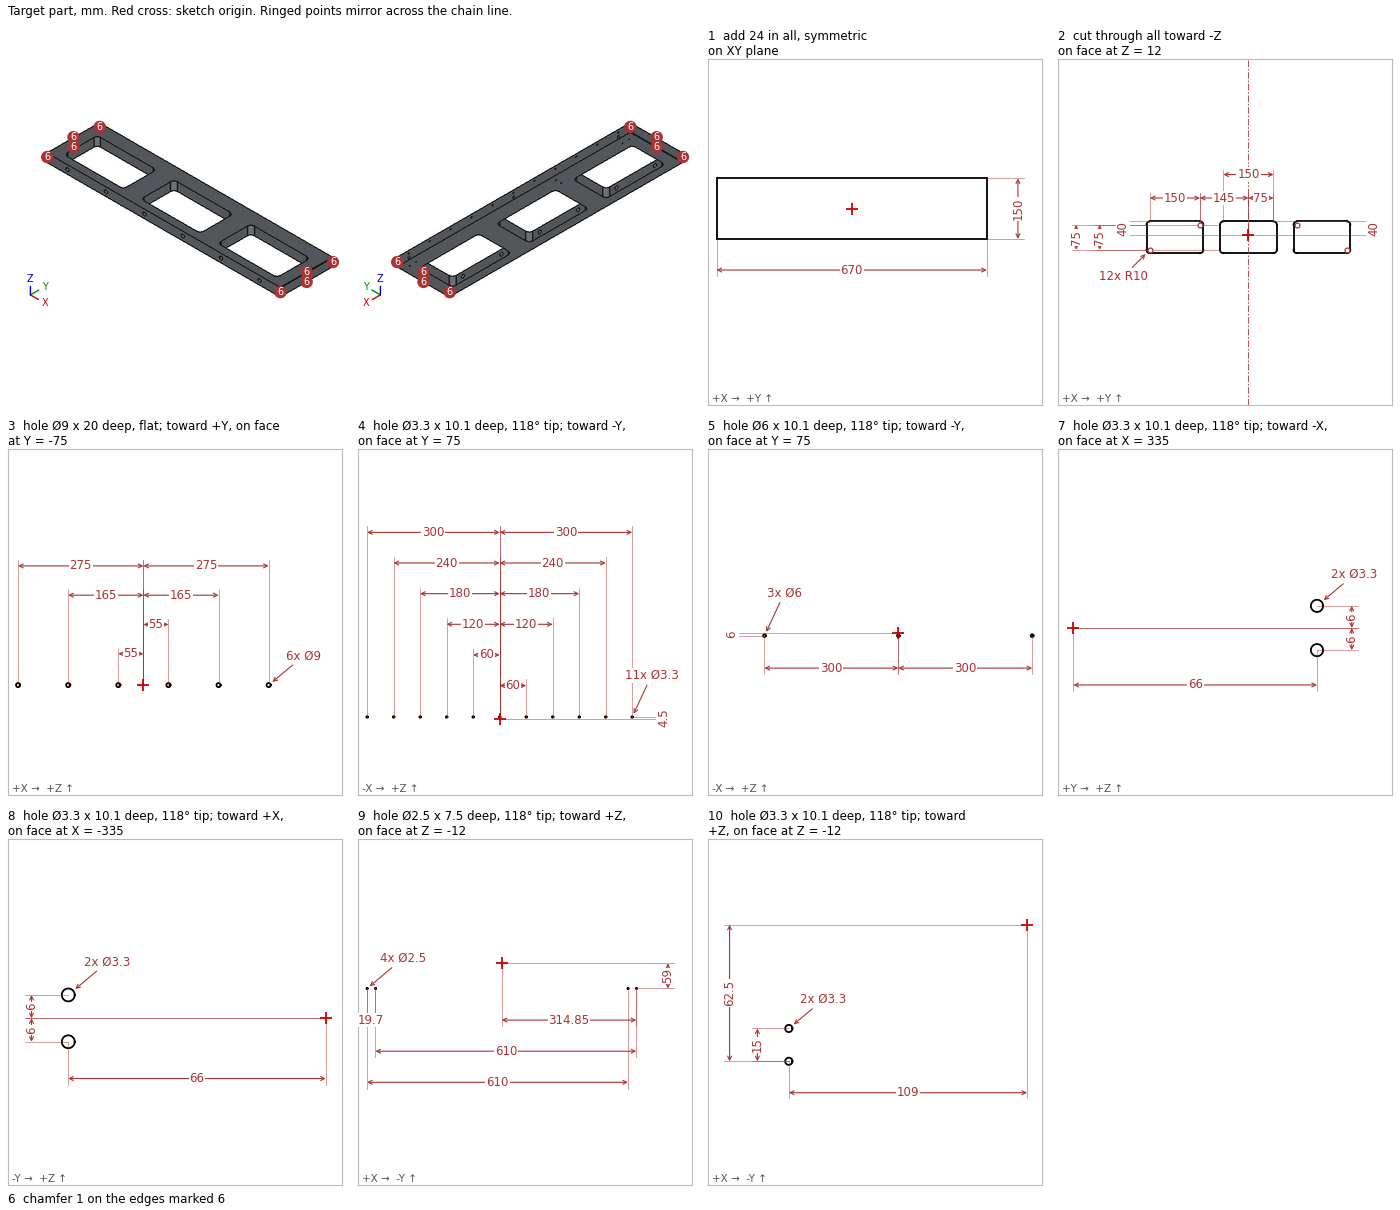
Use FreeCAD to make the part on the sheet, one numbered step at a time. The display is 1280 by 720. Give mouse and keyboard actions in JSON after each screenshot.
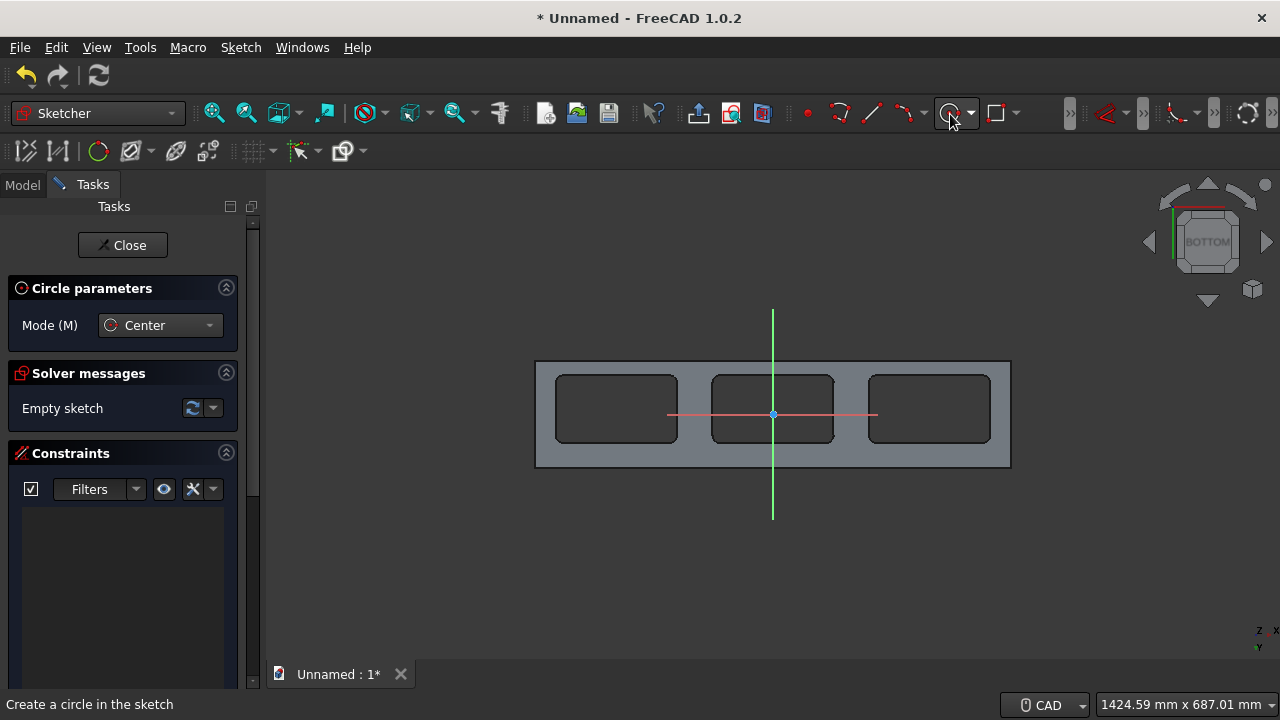
{"action": "scroll", "coordinate": [997, 456], "scroll_direction": "up", "scroll_amount": 17}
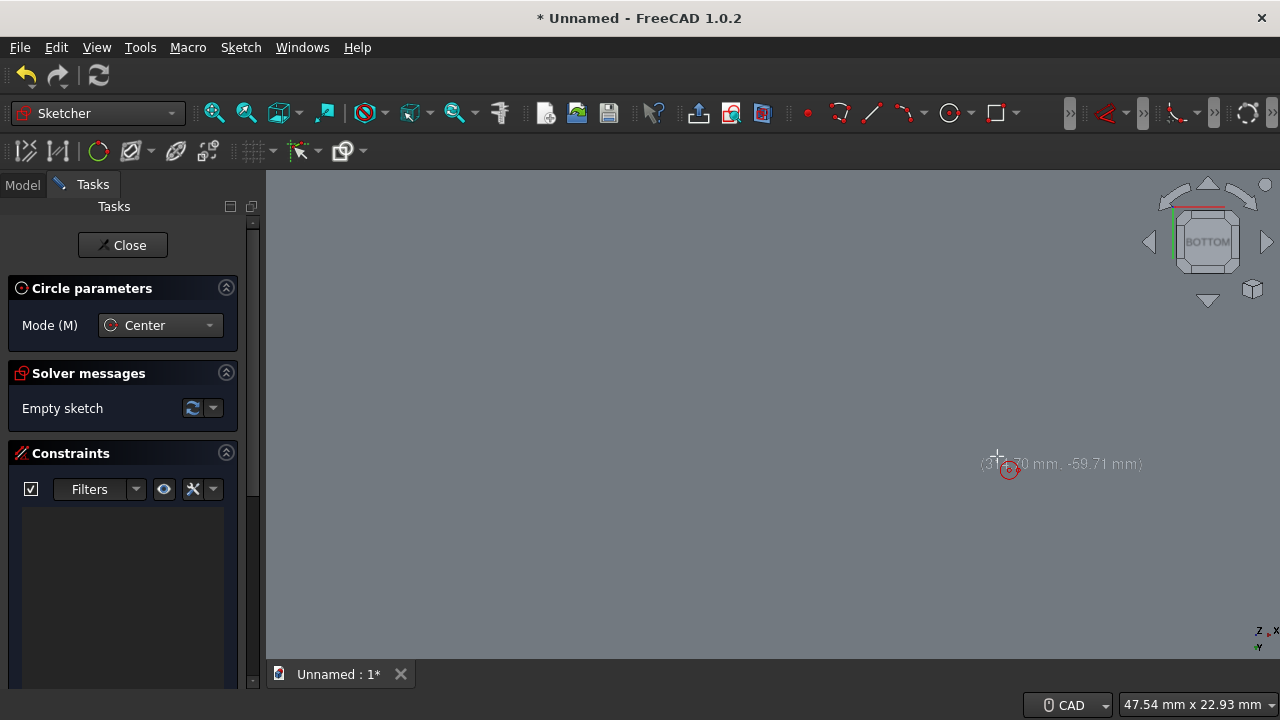
{"action": "scroll", "coordinate": [1042, 445], "scroll_direction": "down", "scroll_amount": 15}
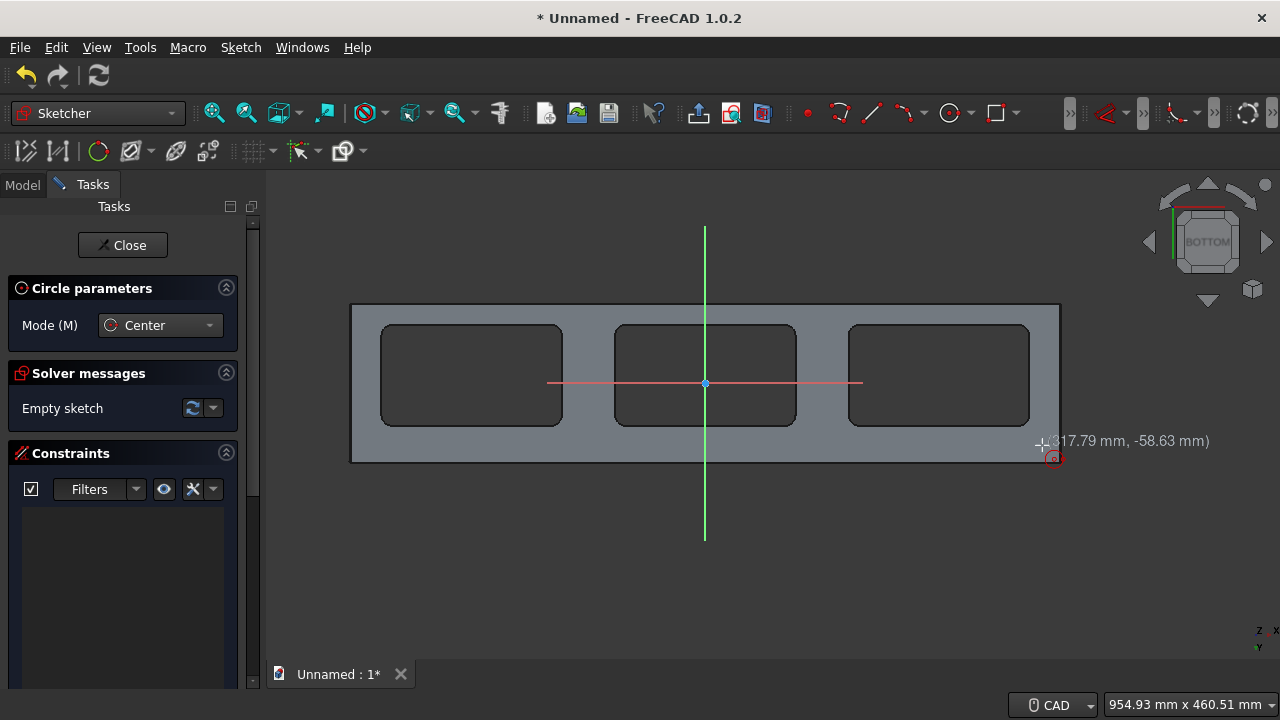
{"action": "left_click", "coordinate": [1040, 446]}
{"action": "mouse_move", "coordinate": [1041, 445]}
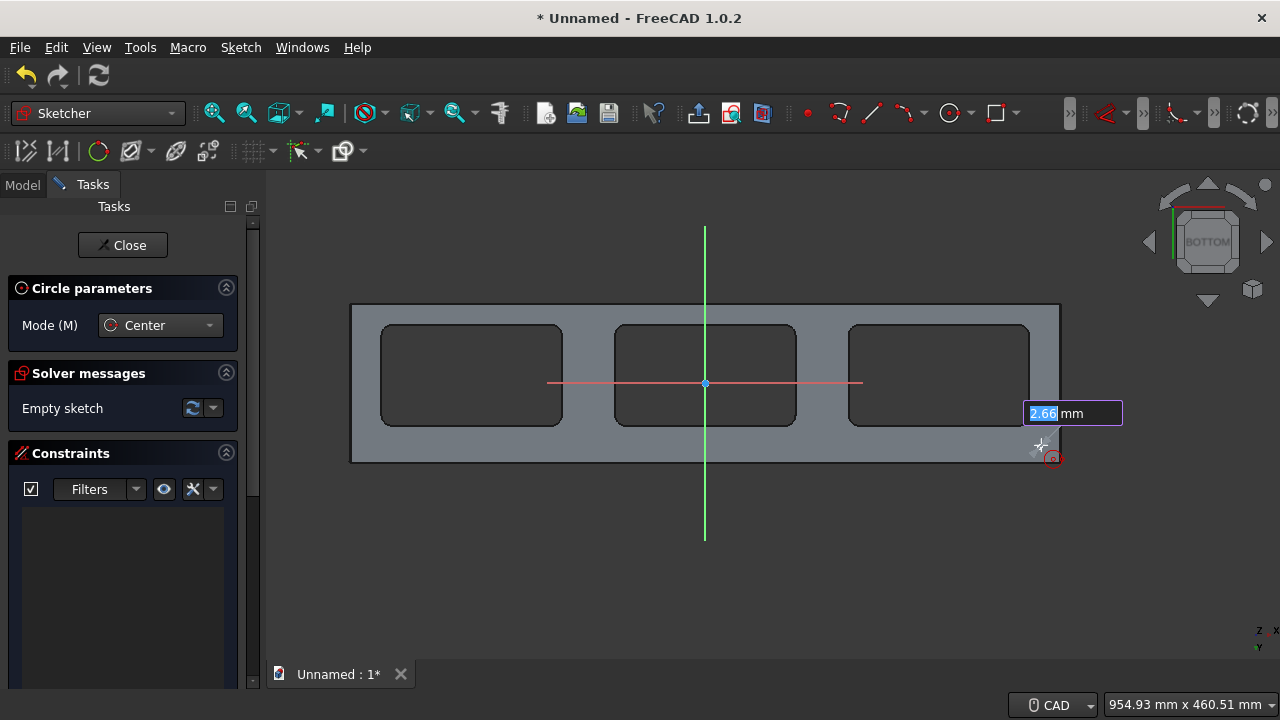
{"action": "type", "text": "2.5"}
{"action": "key", "text": "Return"}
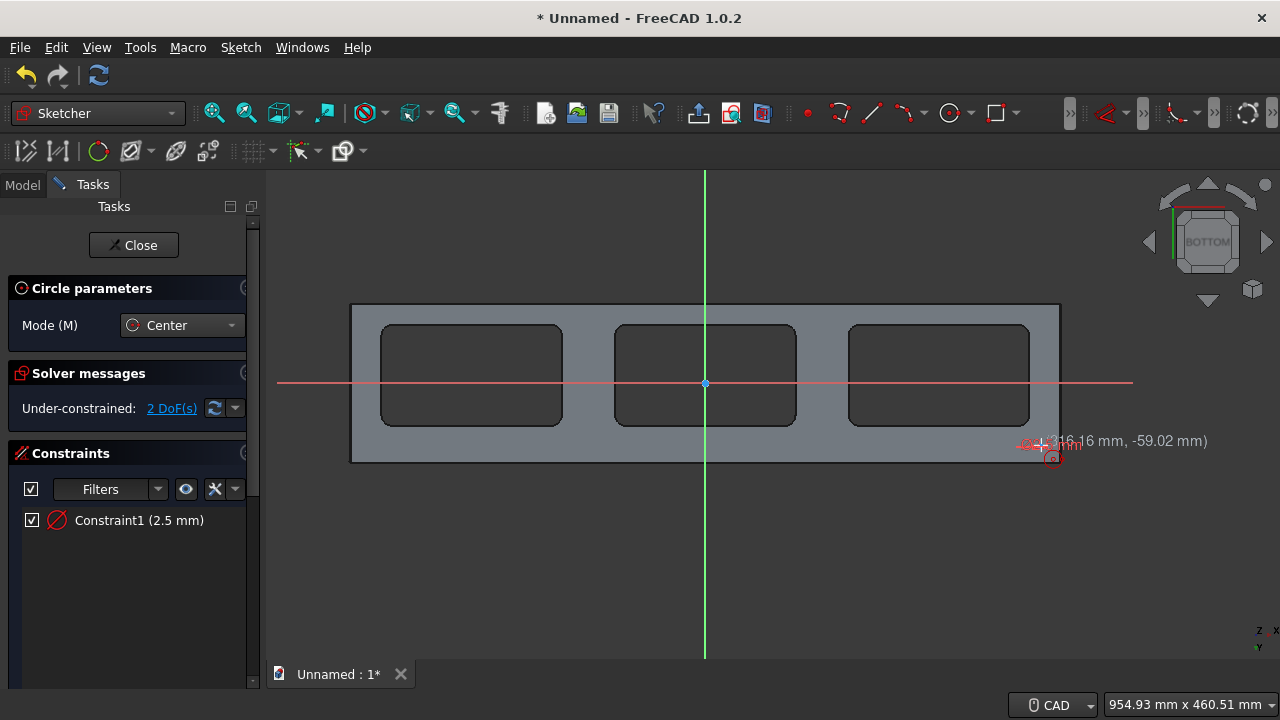
{"action": "scroll", "coordinate": [371, 446], "scroll_direction": "up", "scroll_amount": 15}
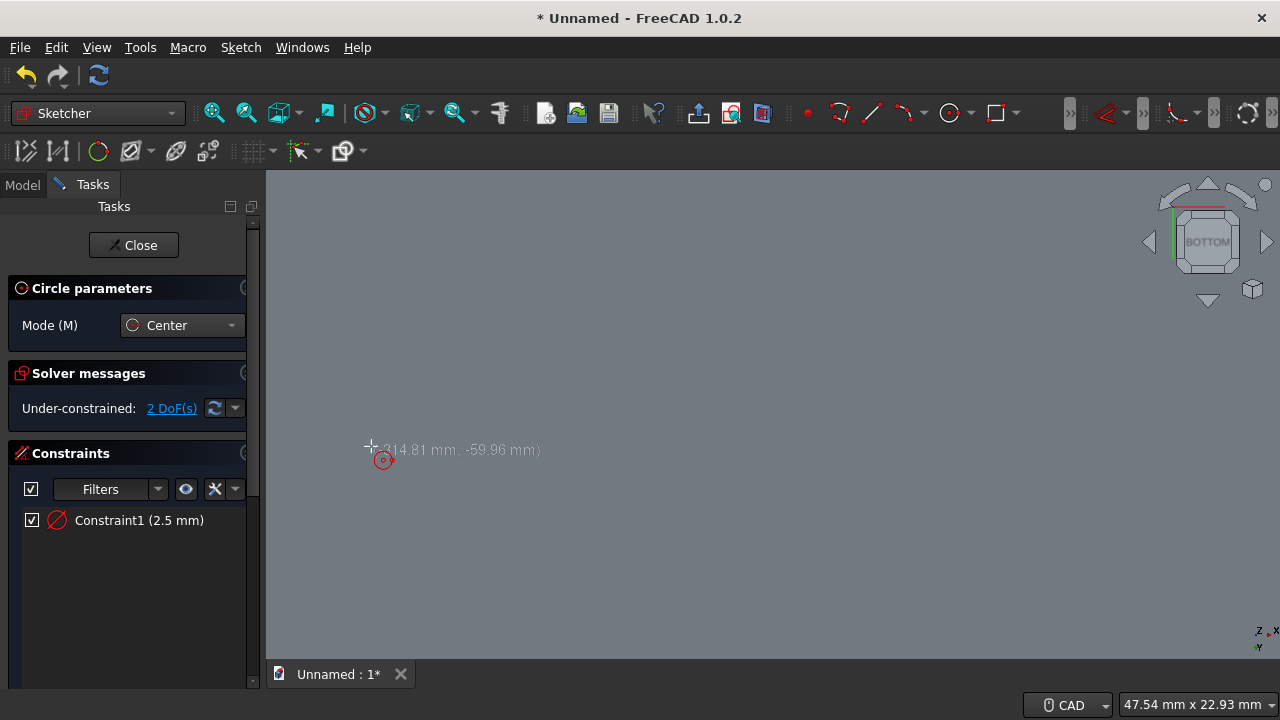
{"action": "scroll", "coordinate": [370, 446], "scroll_direction": "down", "scroll_amount": 15}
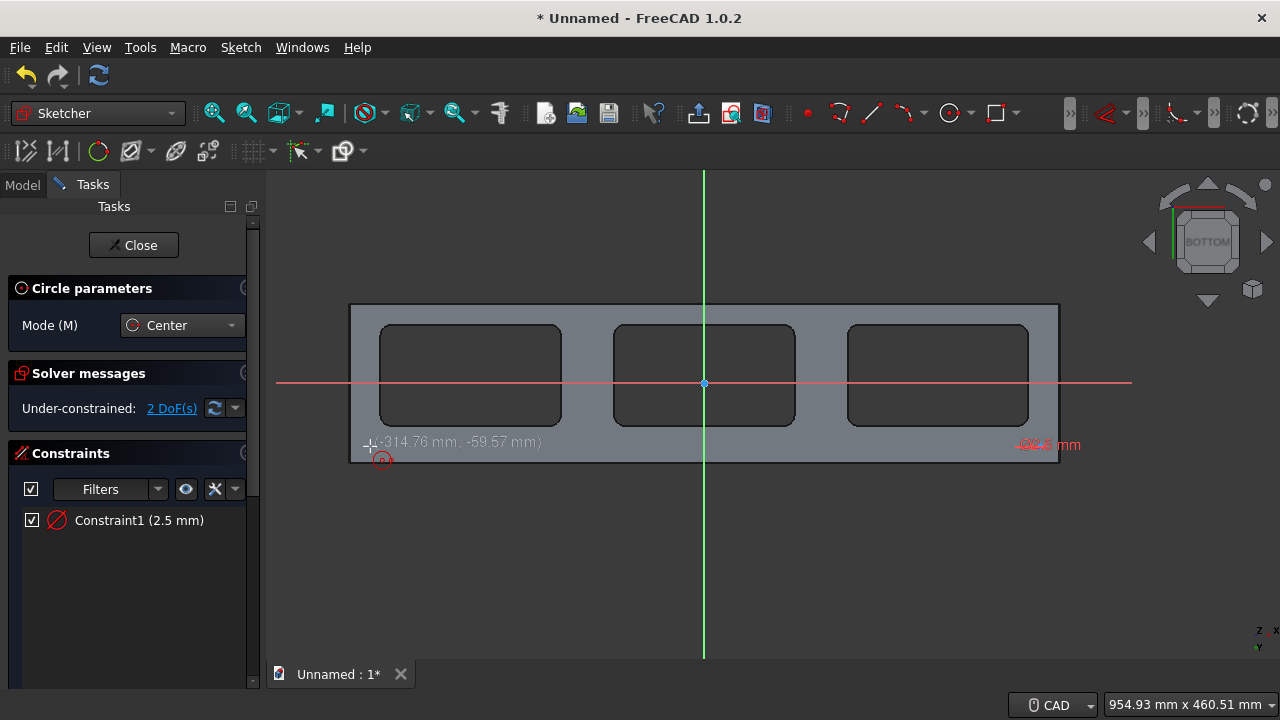
{"action": "left_click", "coordinate": [370, 446]}
{"action": "mouse_move", "coordinate": [371, 445]}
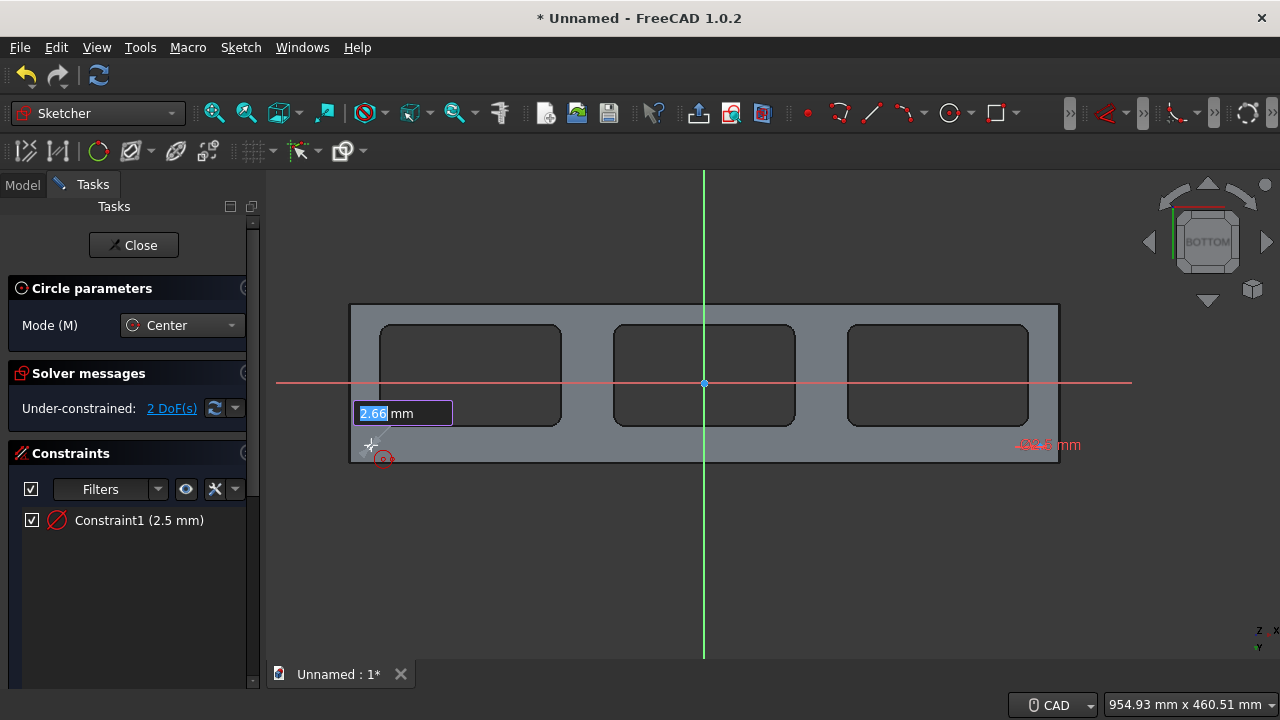
{"action": "type", "text": "2.5"}
{"action": "key", "text": "Return"}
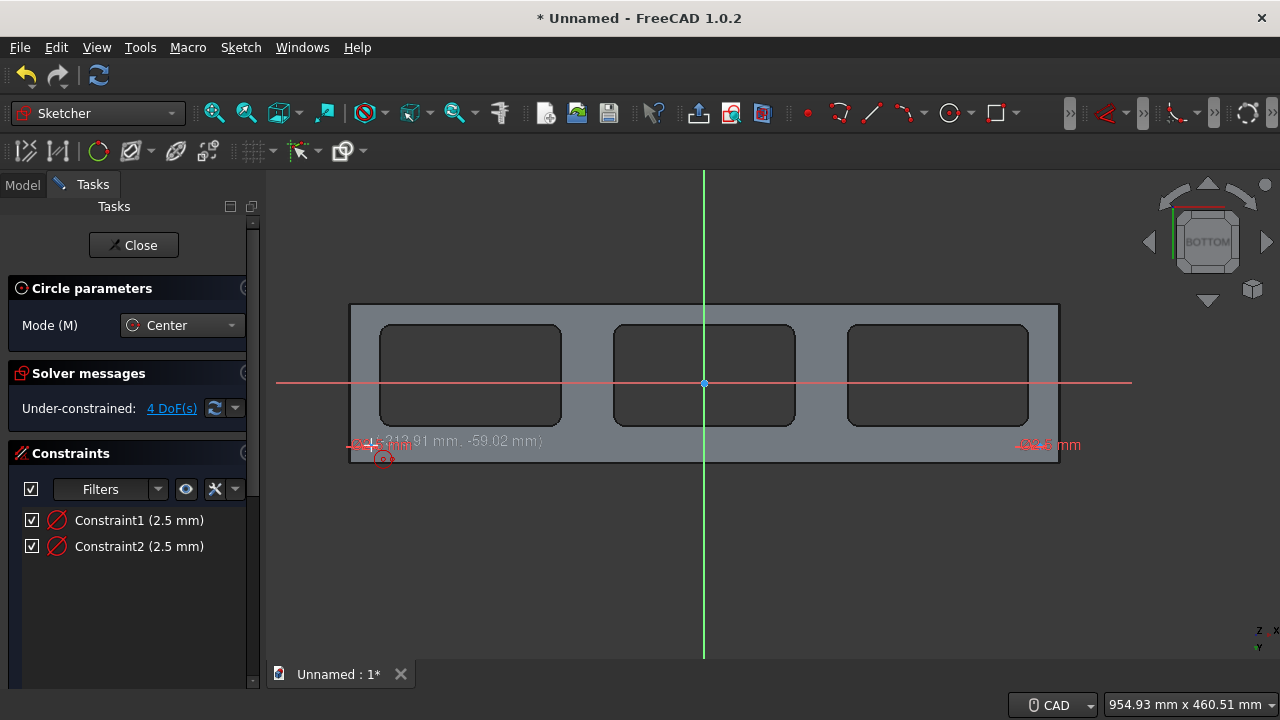
{"action": "scroll", "coordinate": [391, 446], "scroll_direction": "up", "scroll_amount": 15}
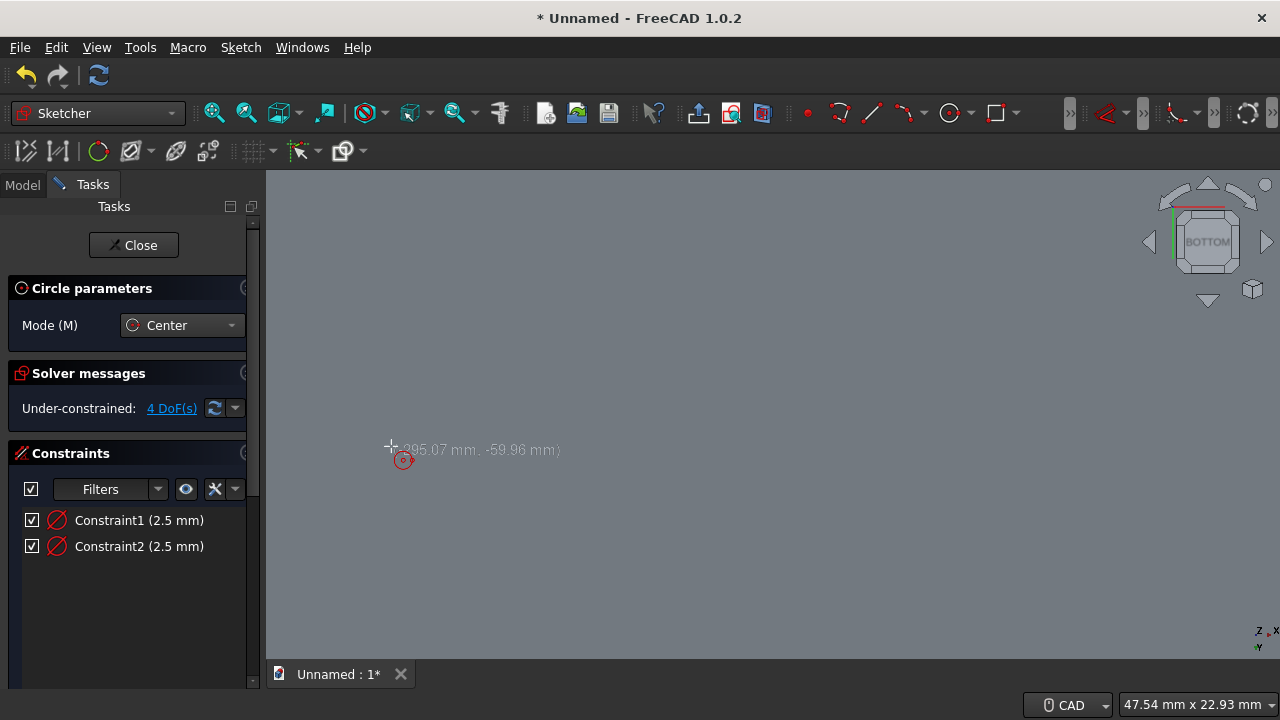
{"action": "scroll", "coordinate": [391, 446], "scroll_direction": "down", "scroll_amount": 15}